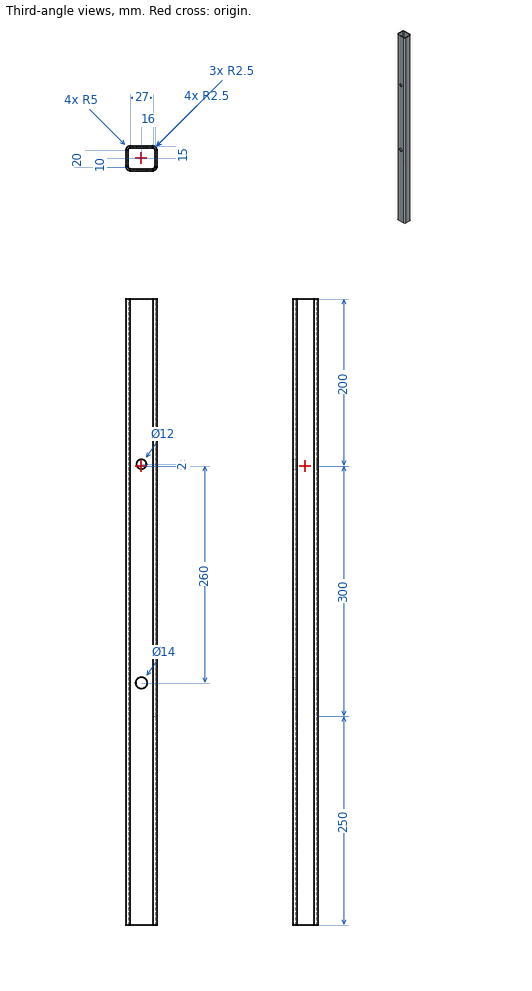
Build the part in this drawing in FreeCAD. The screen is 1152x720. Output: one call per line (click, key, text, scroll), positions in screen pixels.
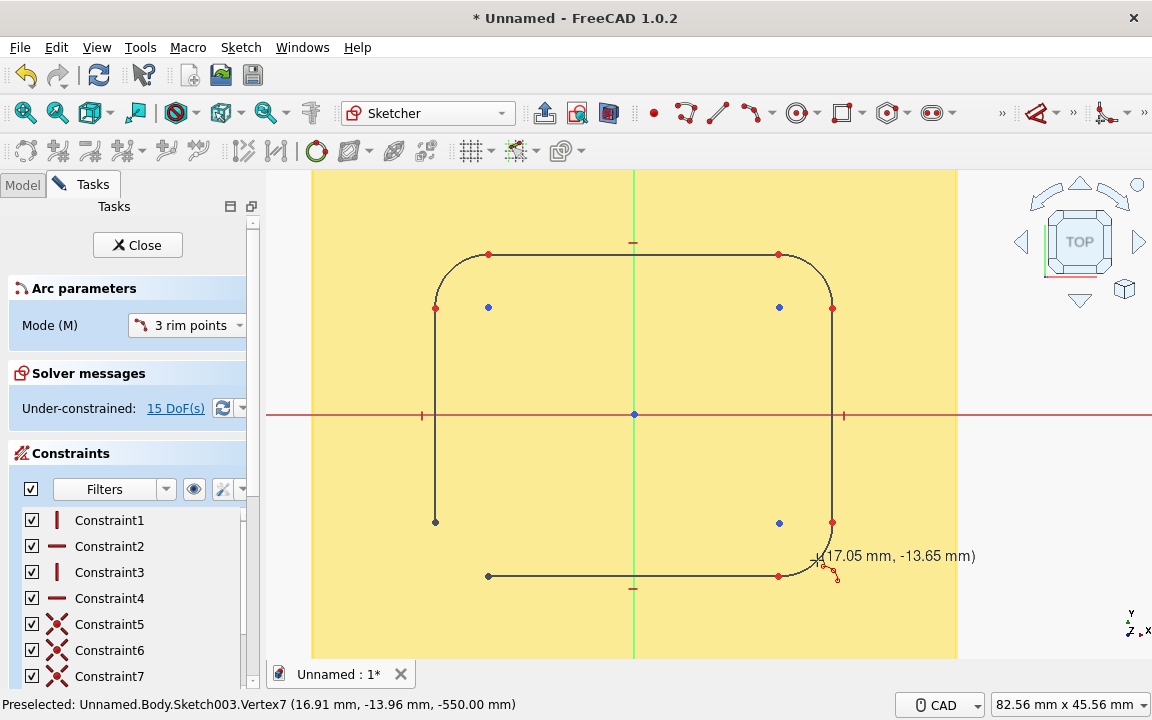
click(489, 576)
click(435, 523)
click(451, 560)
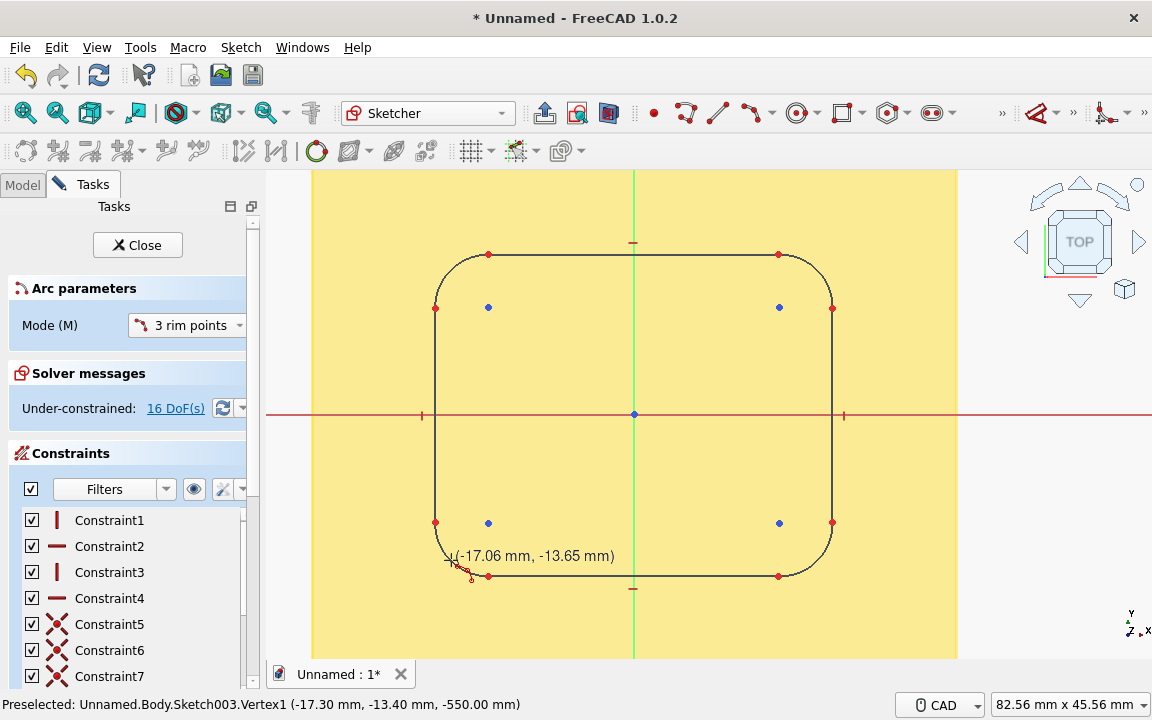
key(g)
key(m)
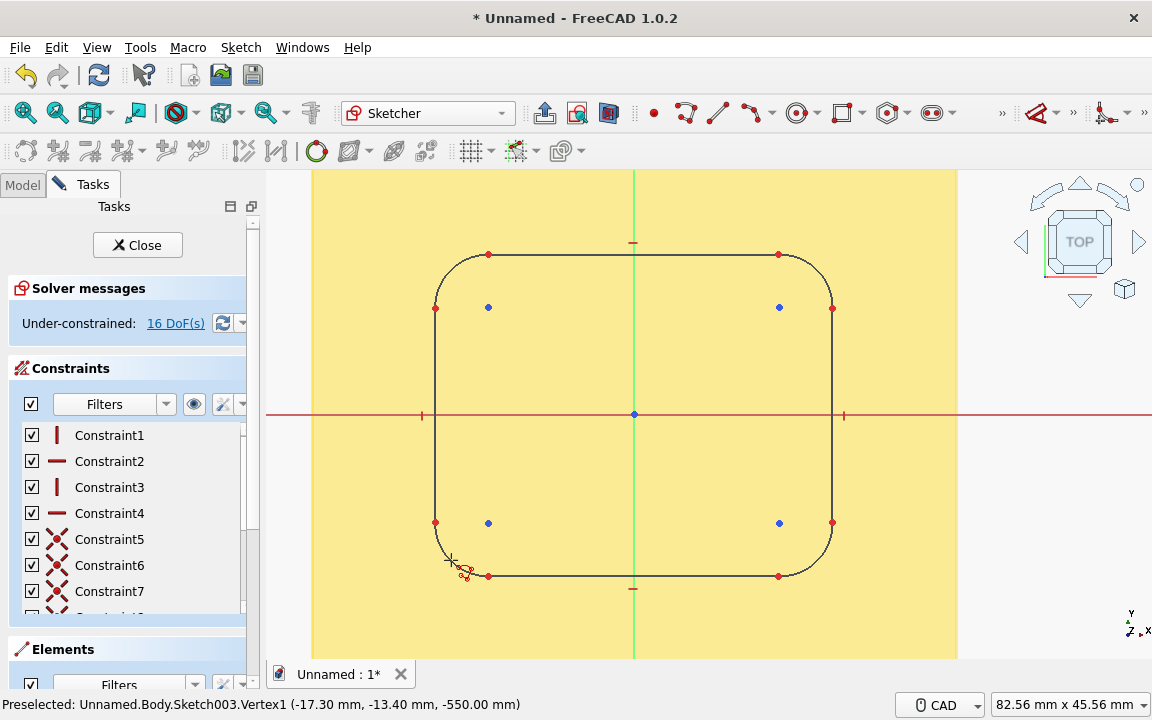
click(489, 549)
click(806, 549)
click(806, 307)
right_click(806, 307)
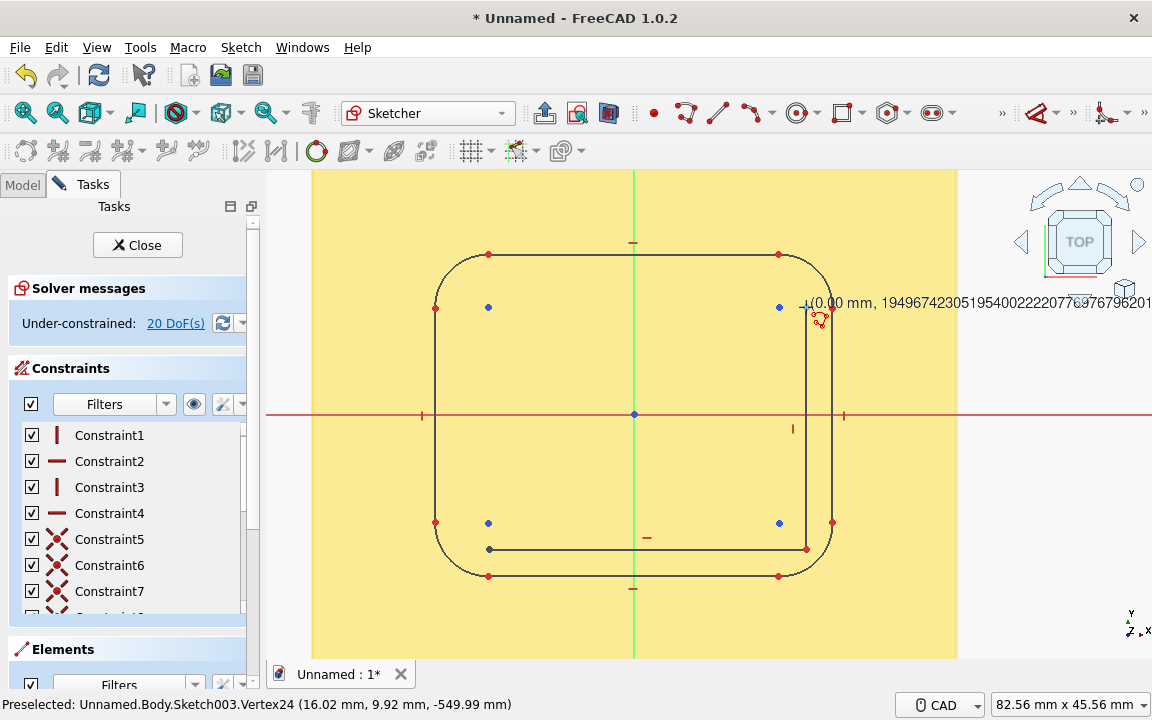
key(g)
key(l)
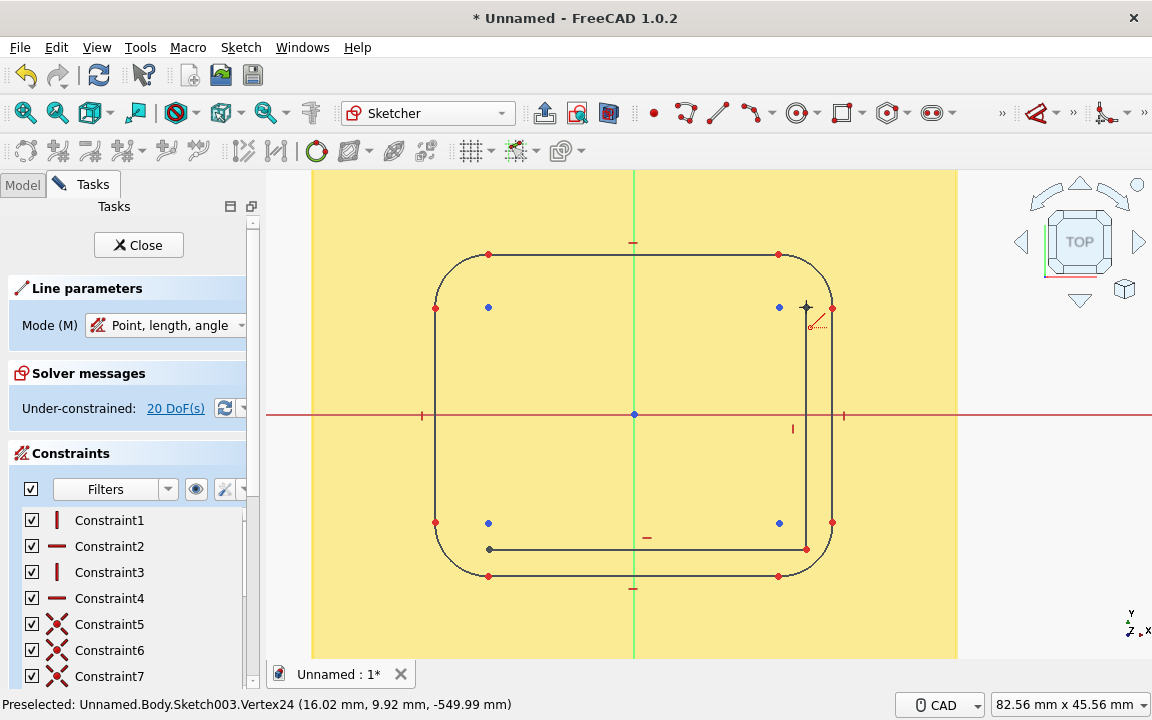
click(779, 280)
click(489, 280)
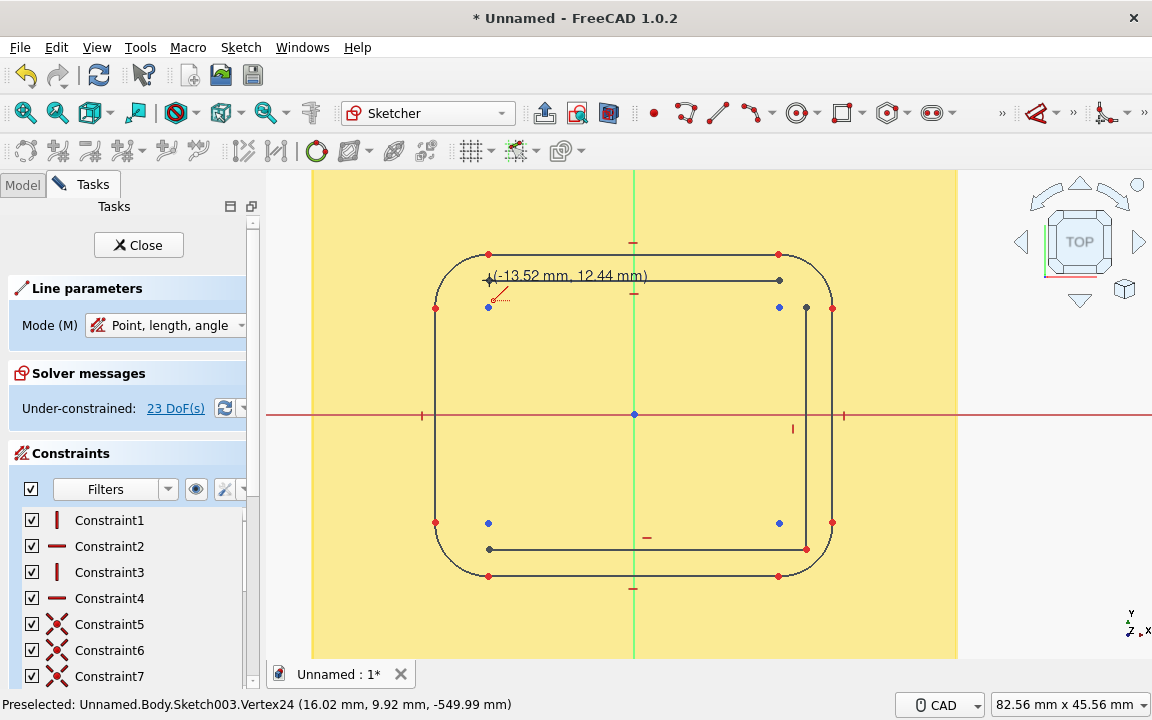
click(462, 307)
click(462, 522)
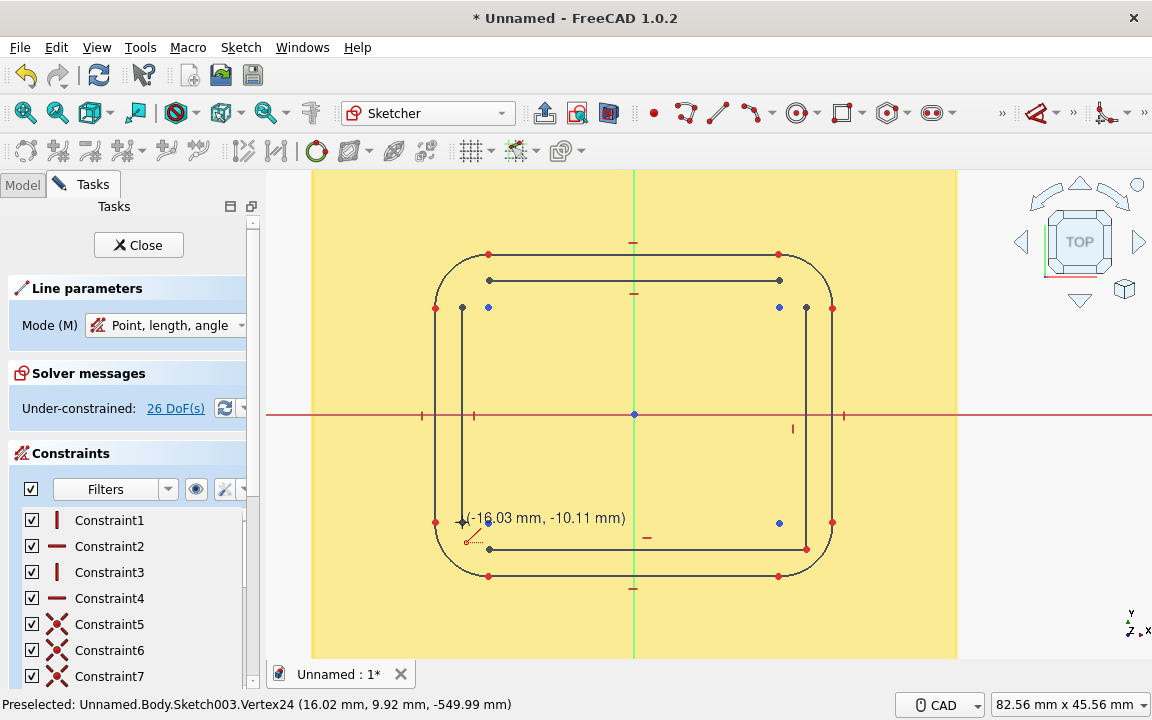
key(g)
key(3)
key(a)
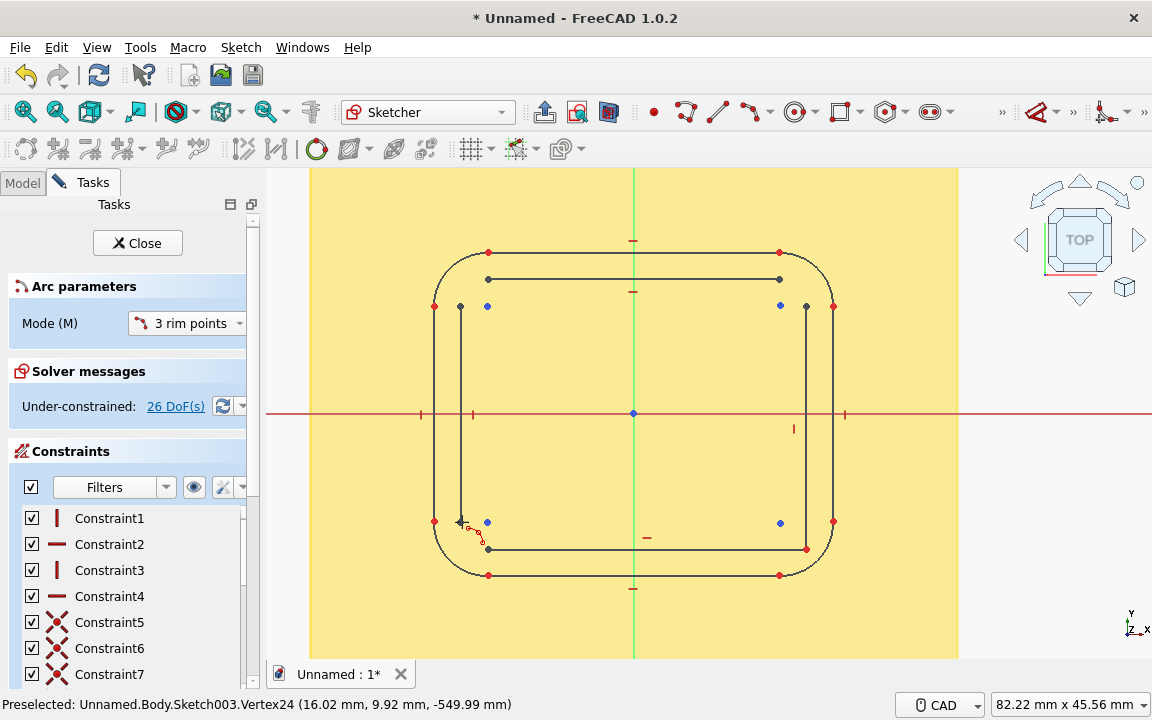
click(806, 307)
click(779, 279)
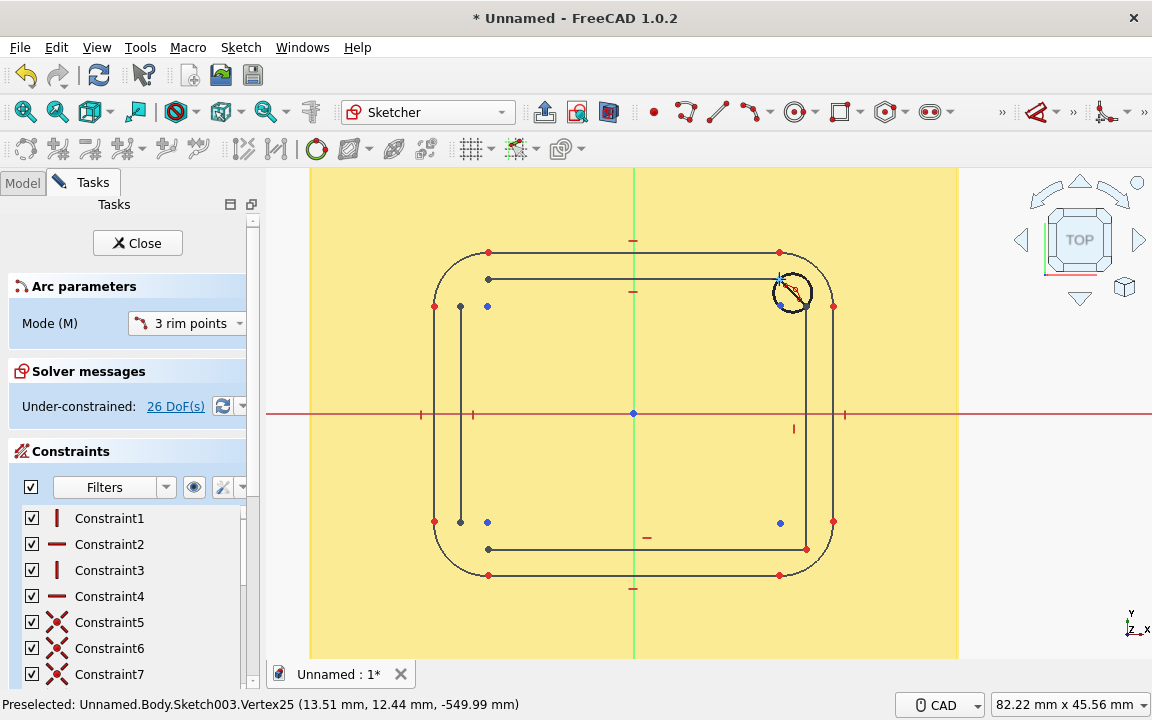
scroll(798, 287, up, 4)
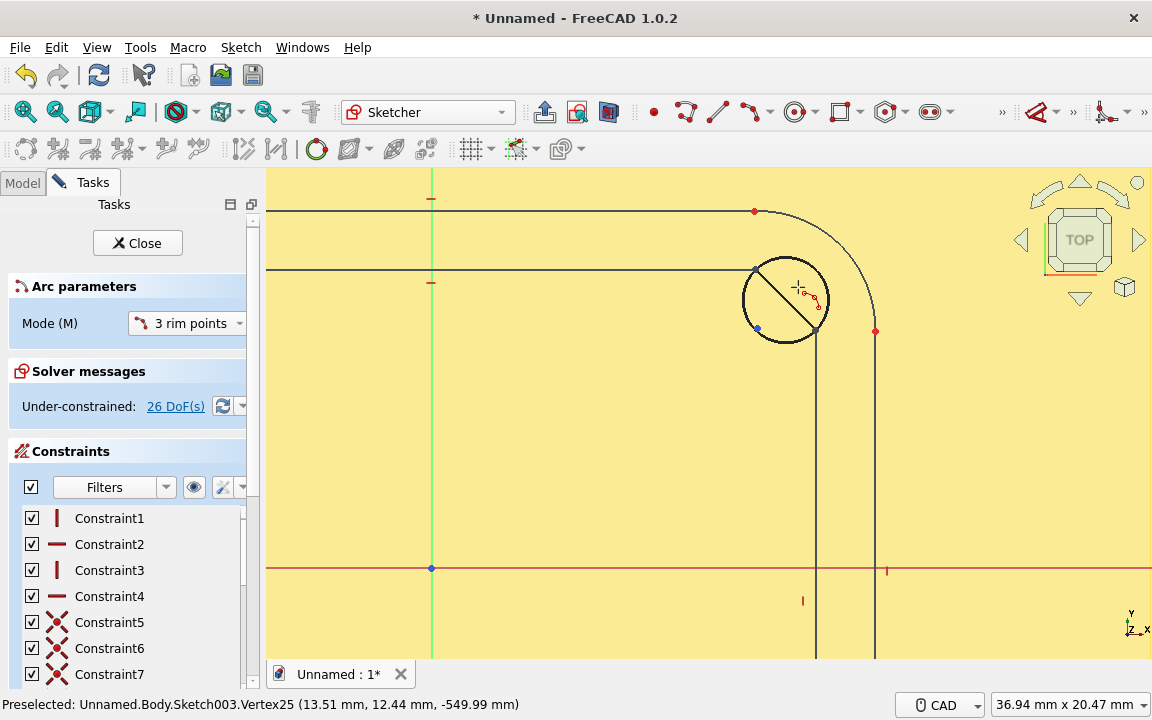
click(798, 286)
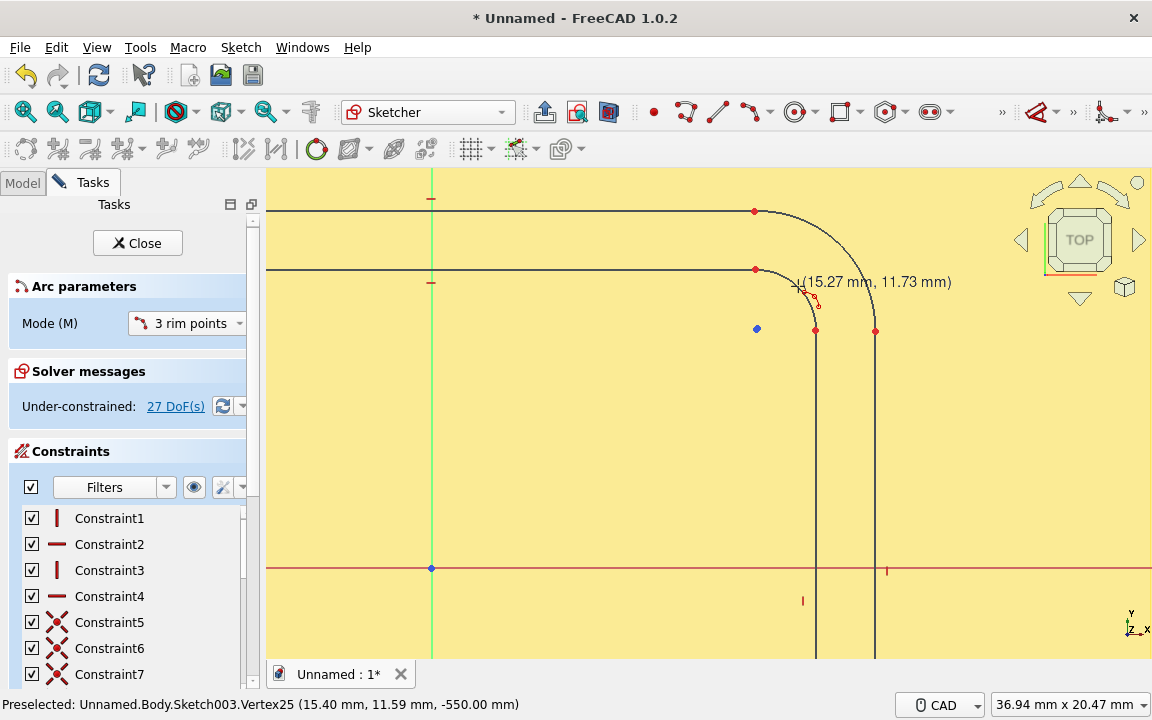
scroll(811, 287, down, 4)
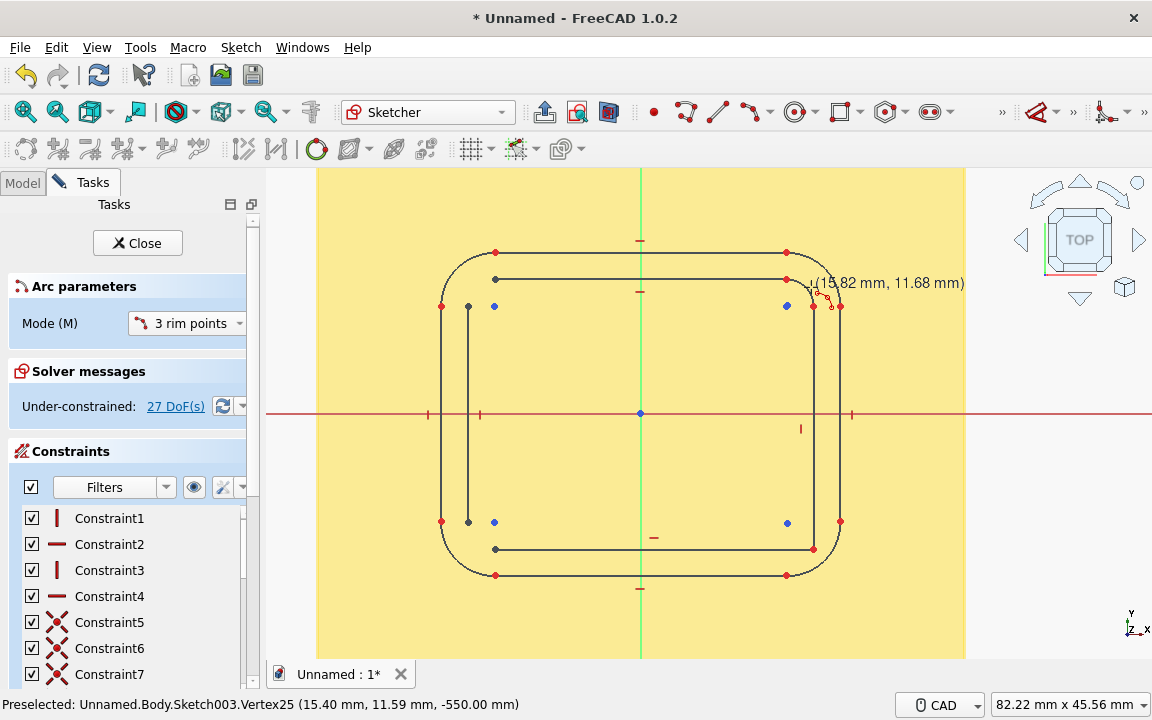
click(495, 279)
click(468, 307)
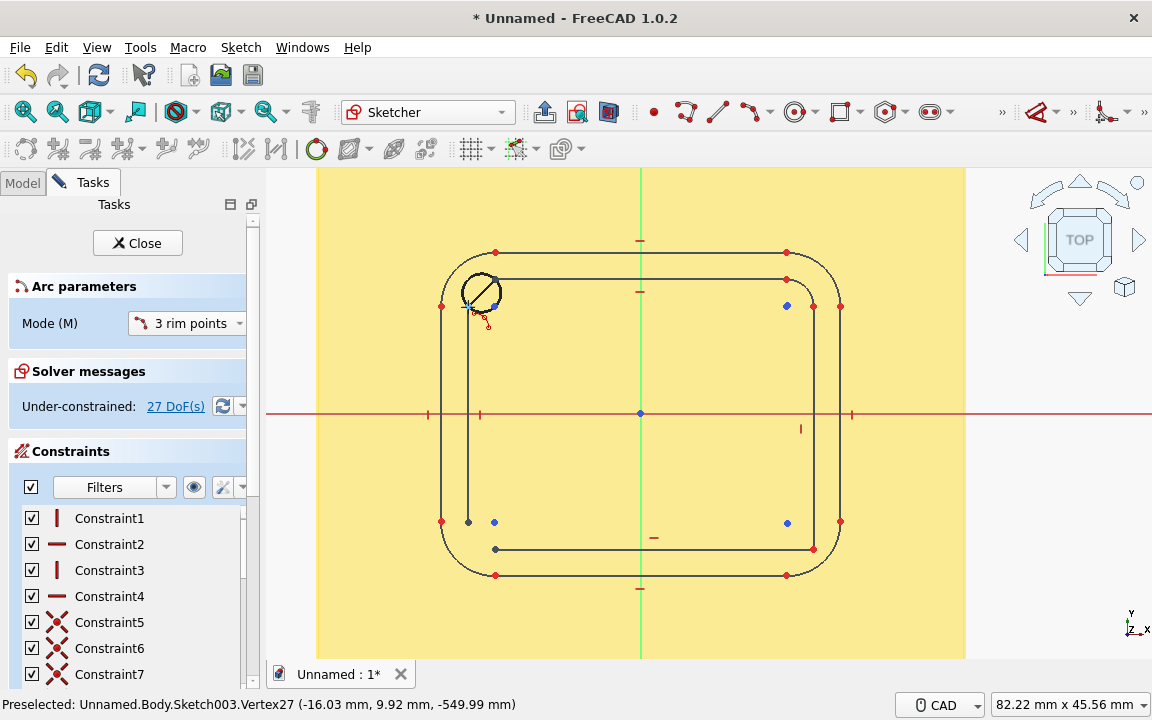
scroll(476, 287, up, 4)